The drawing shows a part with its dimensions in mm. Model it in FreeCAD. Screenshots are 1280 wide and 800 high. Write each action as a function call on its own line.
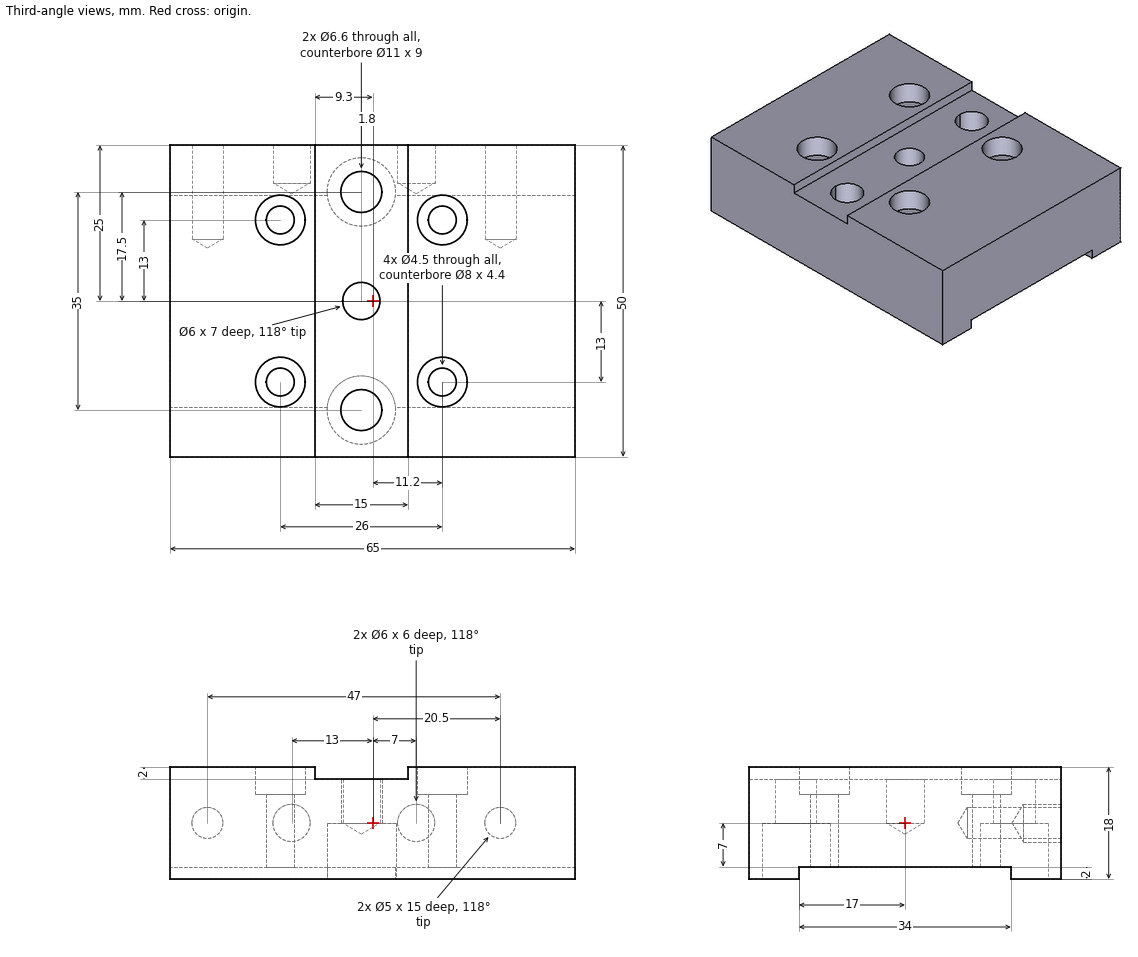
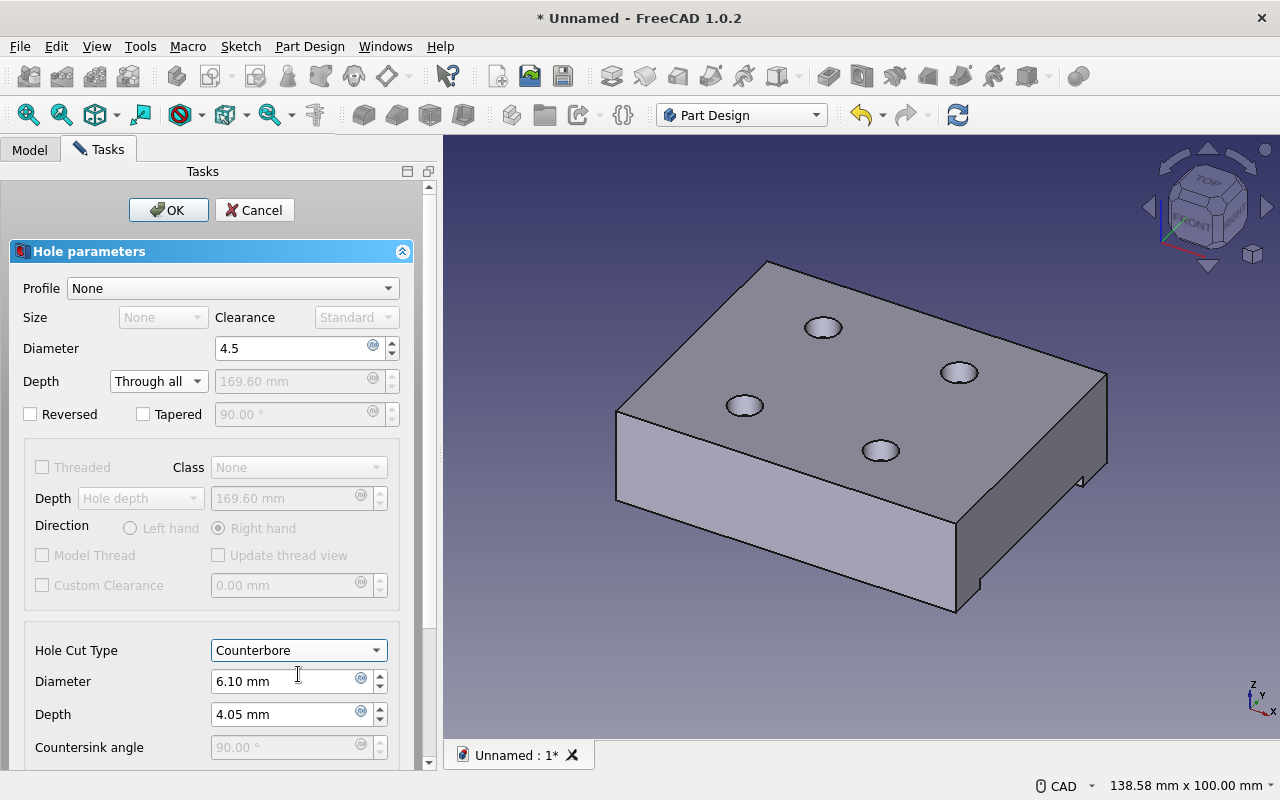
triple_click(292, 682)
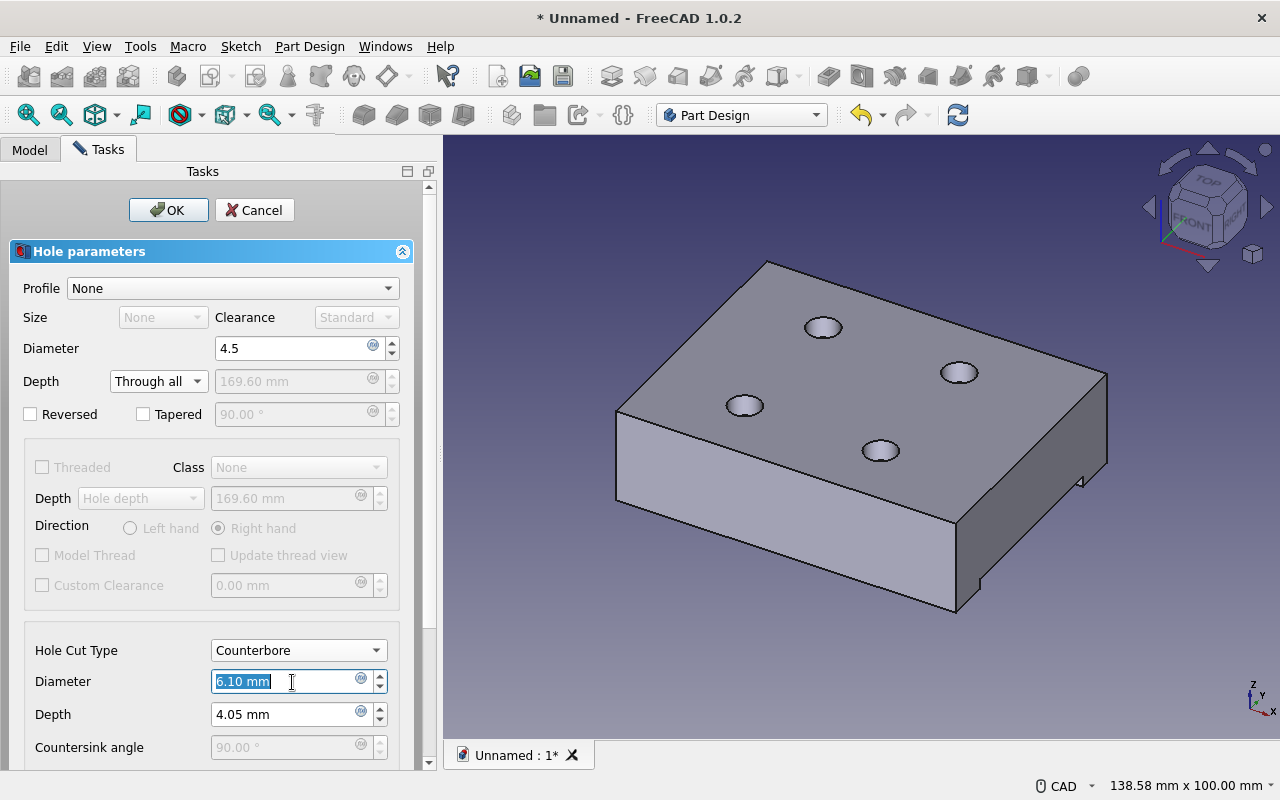
text(8)
key(Tab)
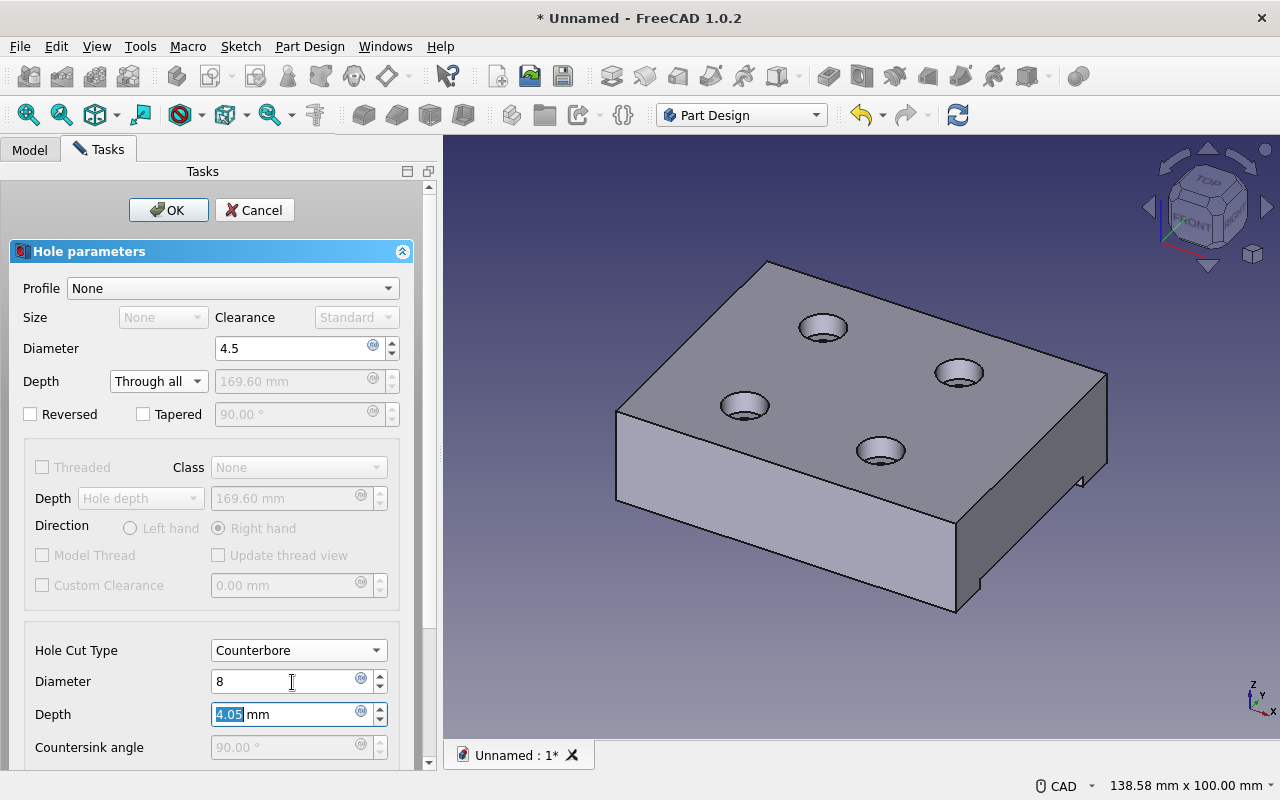
text(4.4)
key(Tab)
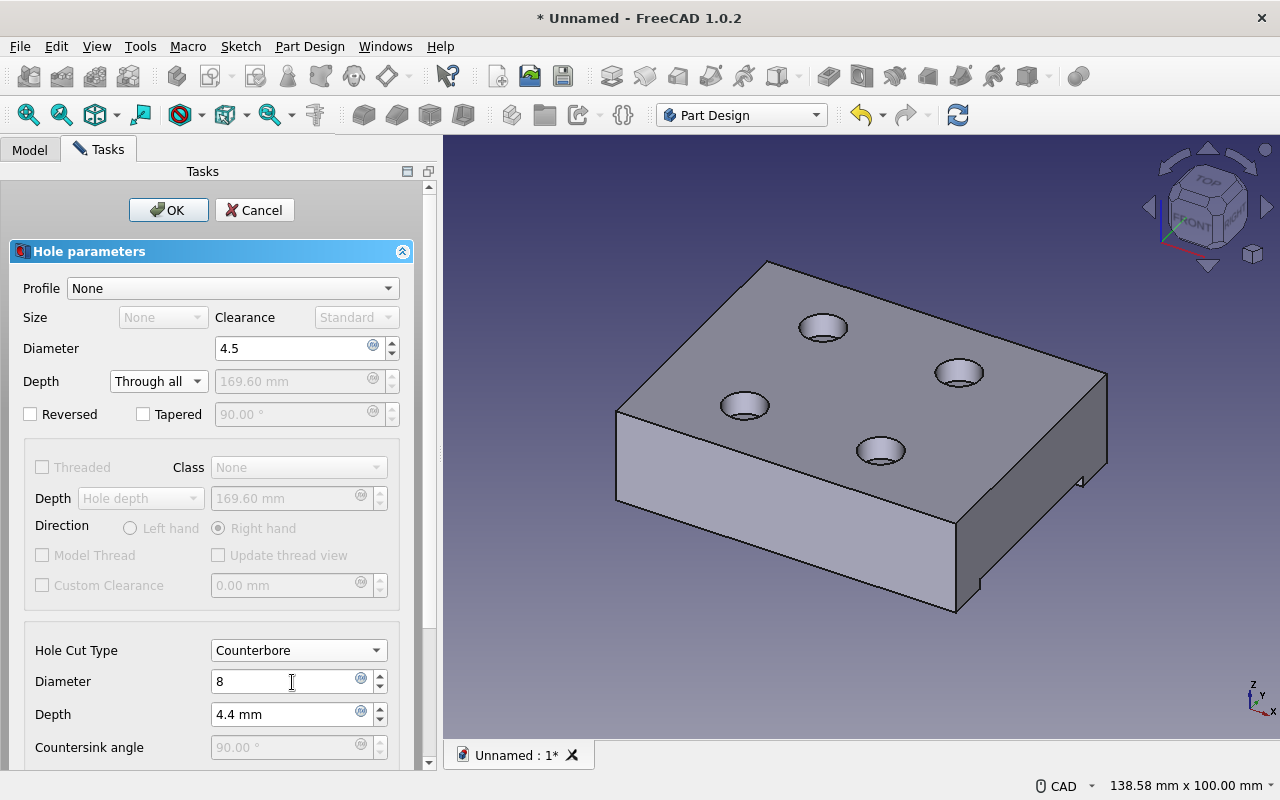
click(169, 210)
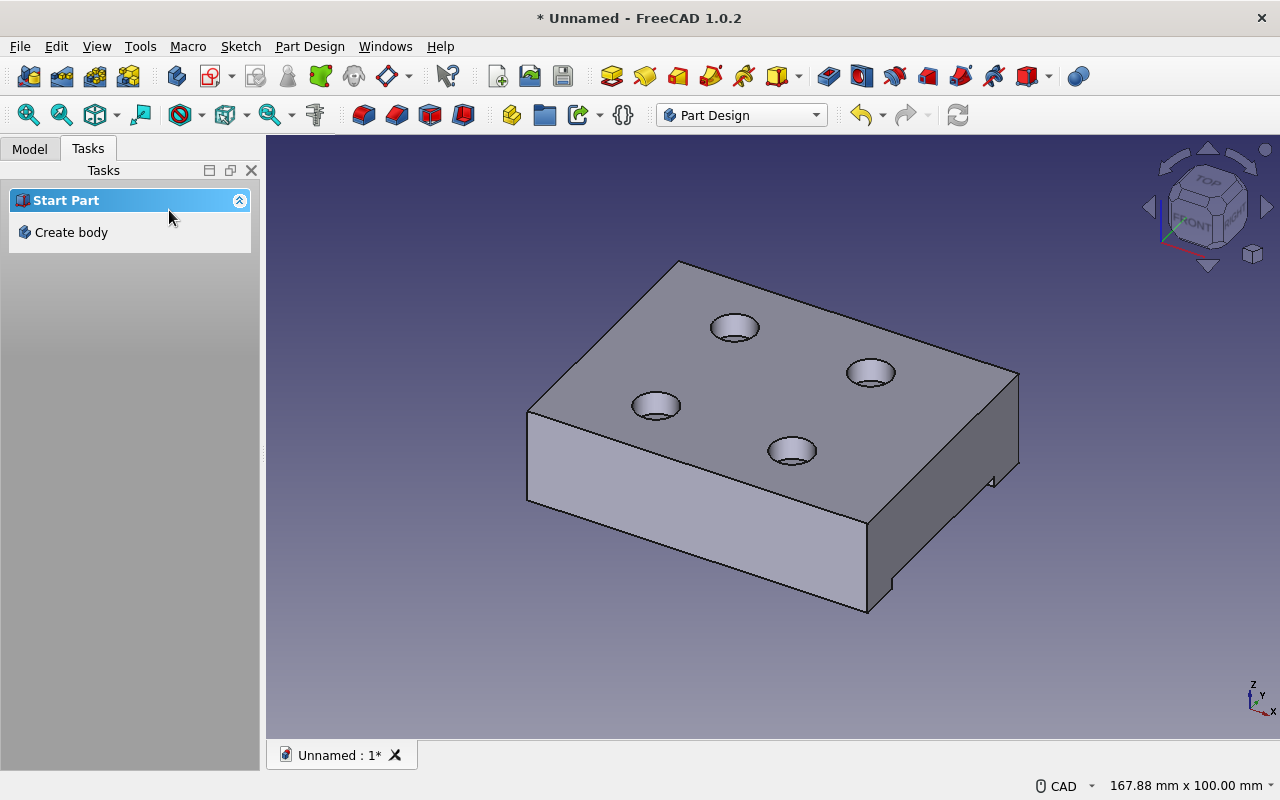
click(773, 391)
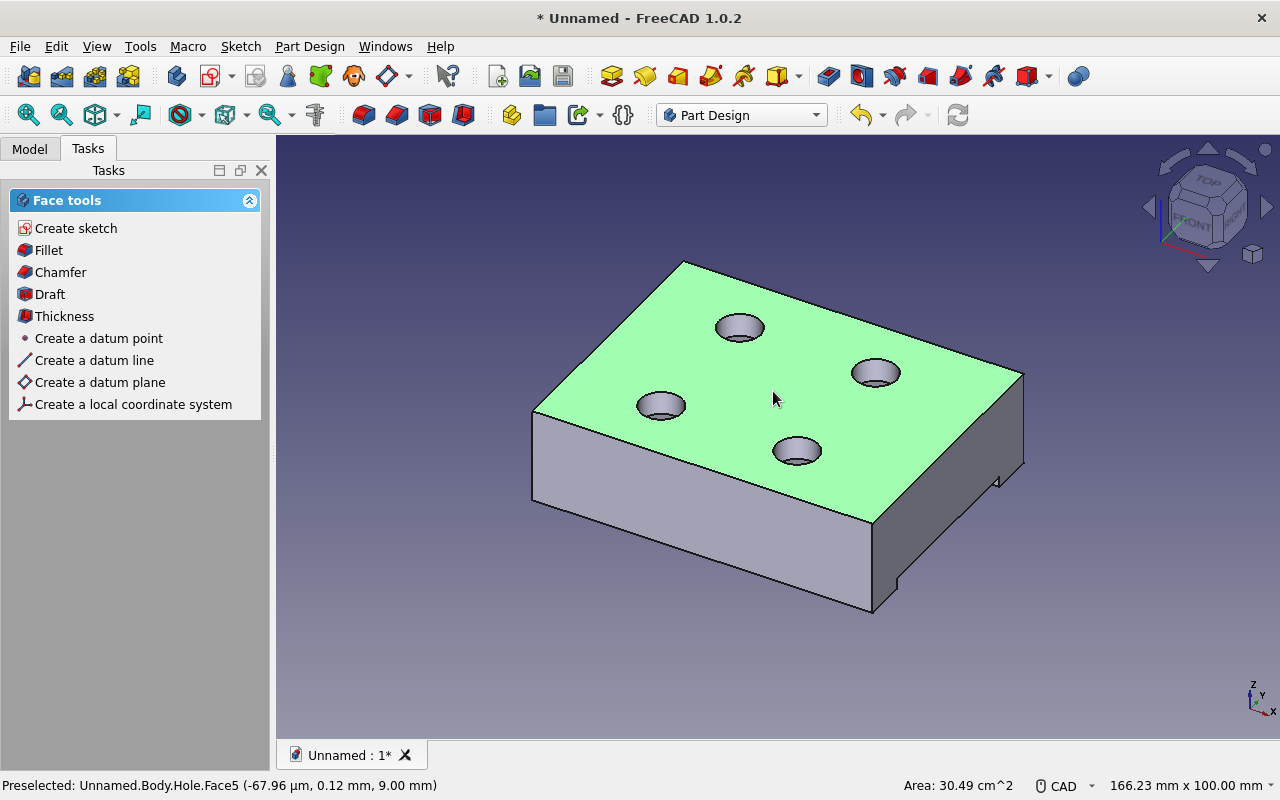
click(210, 76)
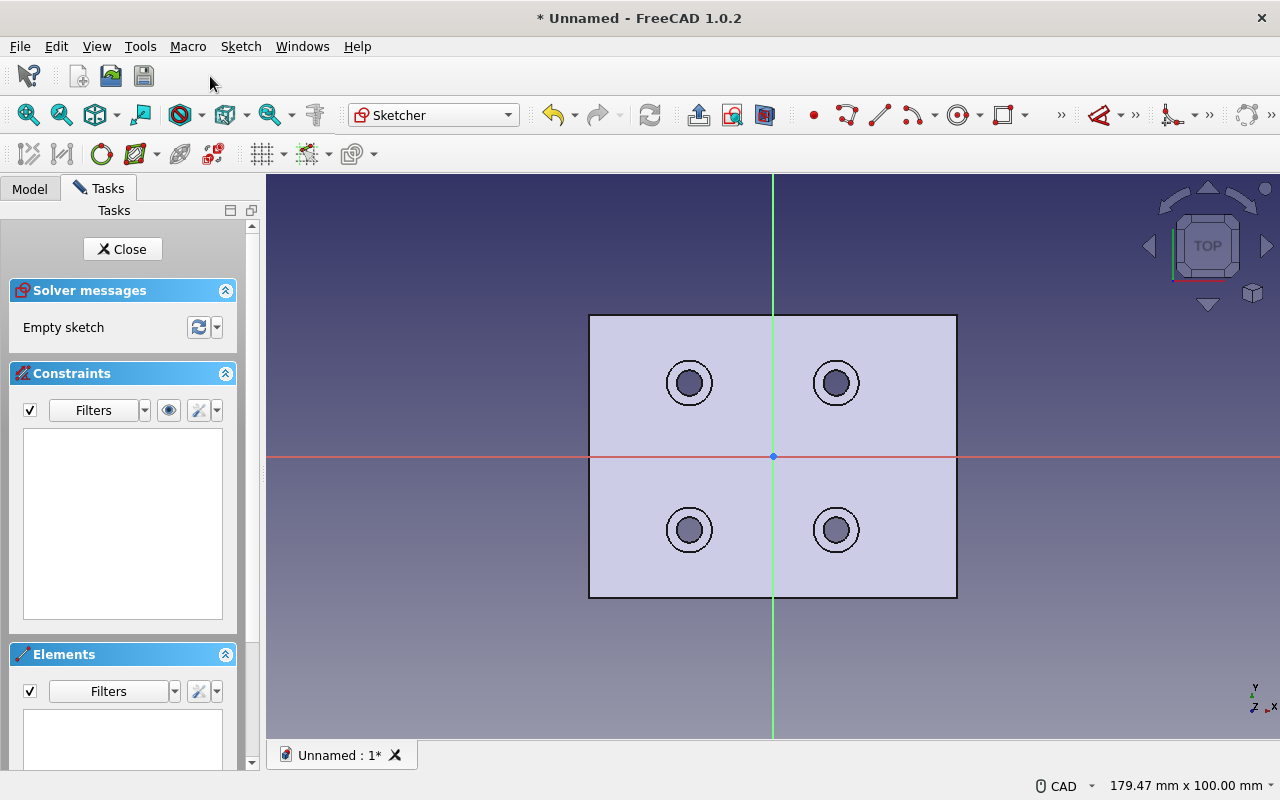
key(g)
key(r)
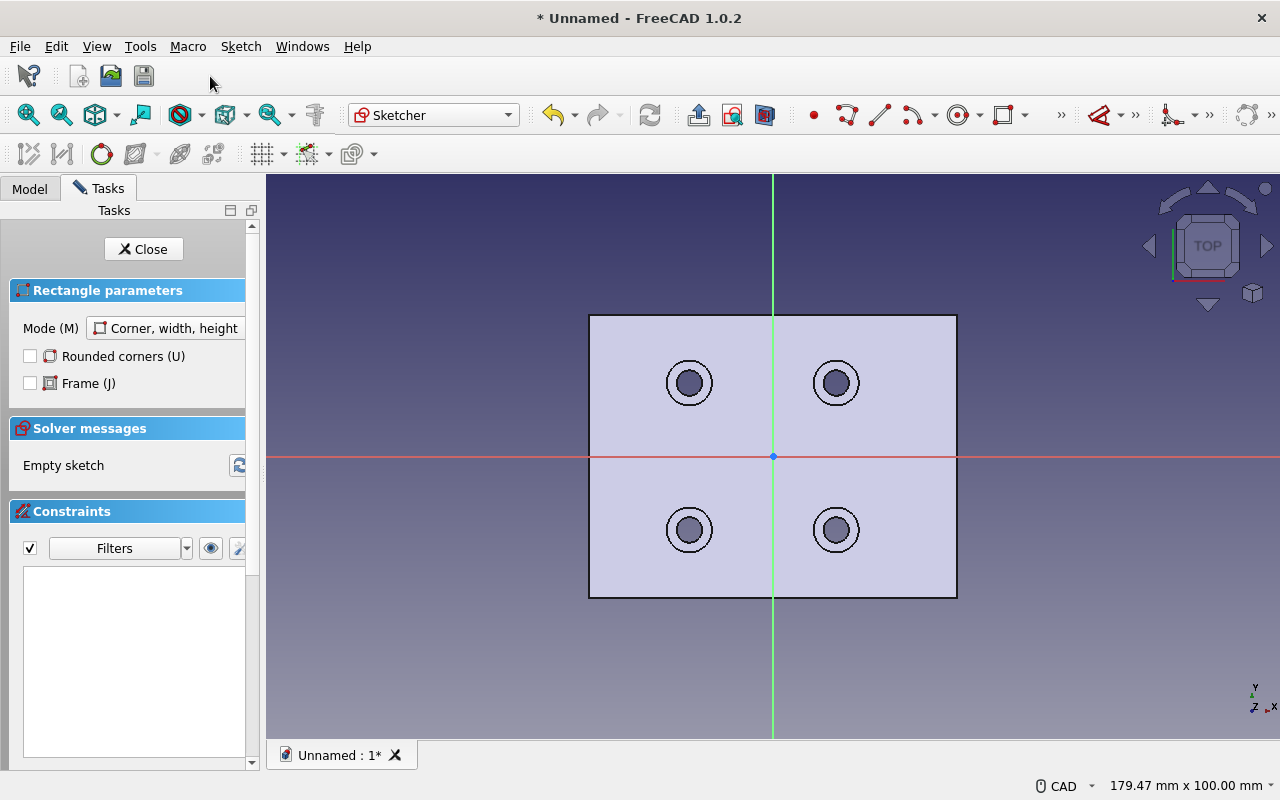
click(720, 315)
move(805, 598)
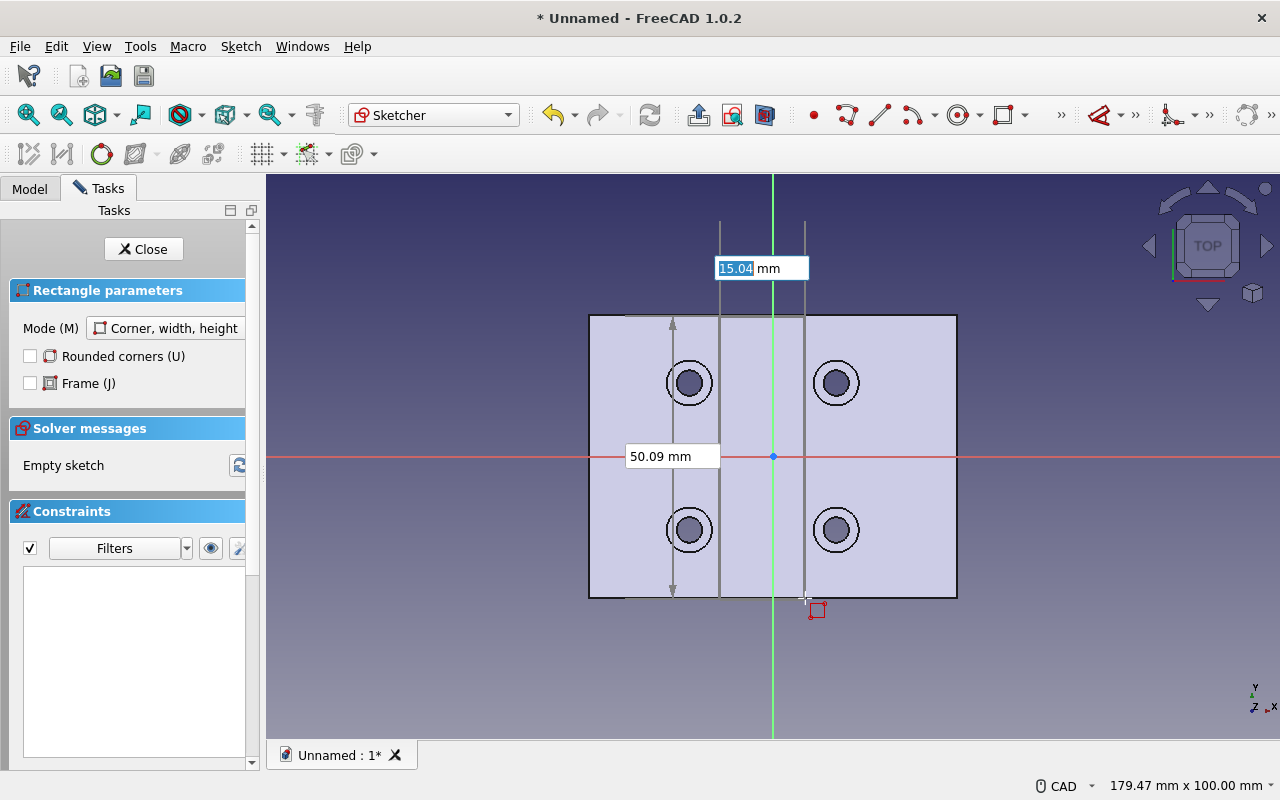
text(15)
key(Tab)
text(50)
key(Return)
key(Escape)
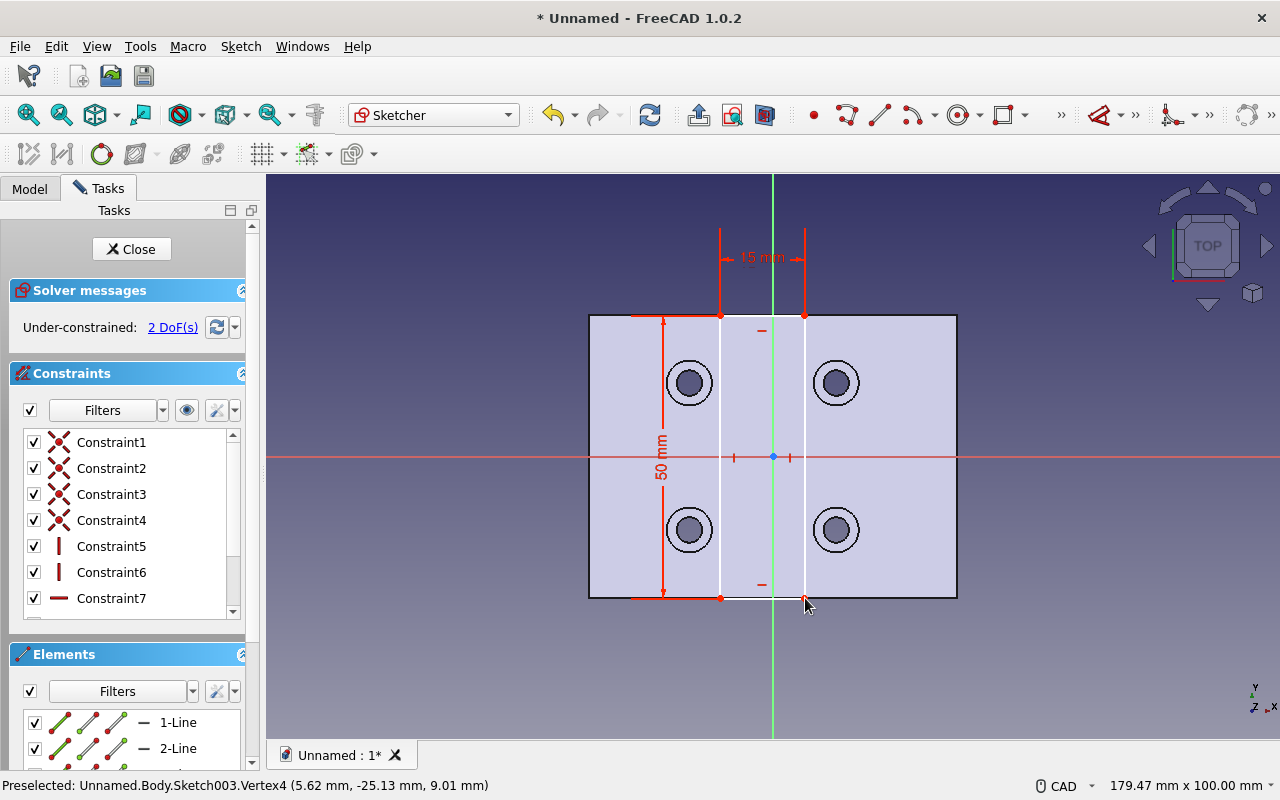
key(d)